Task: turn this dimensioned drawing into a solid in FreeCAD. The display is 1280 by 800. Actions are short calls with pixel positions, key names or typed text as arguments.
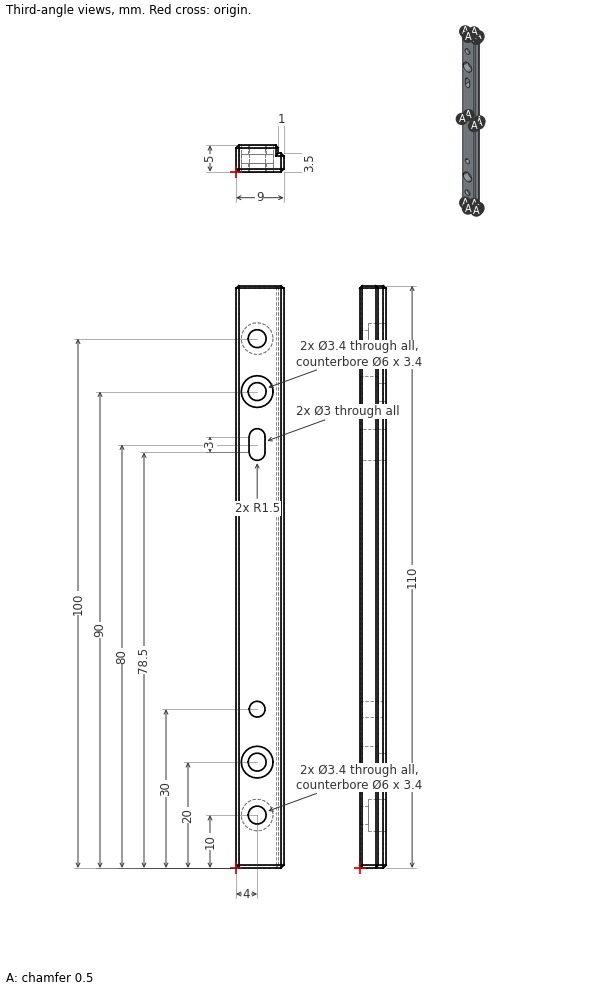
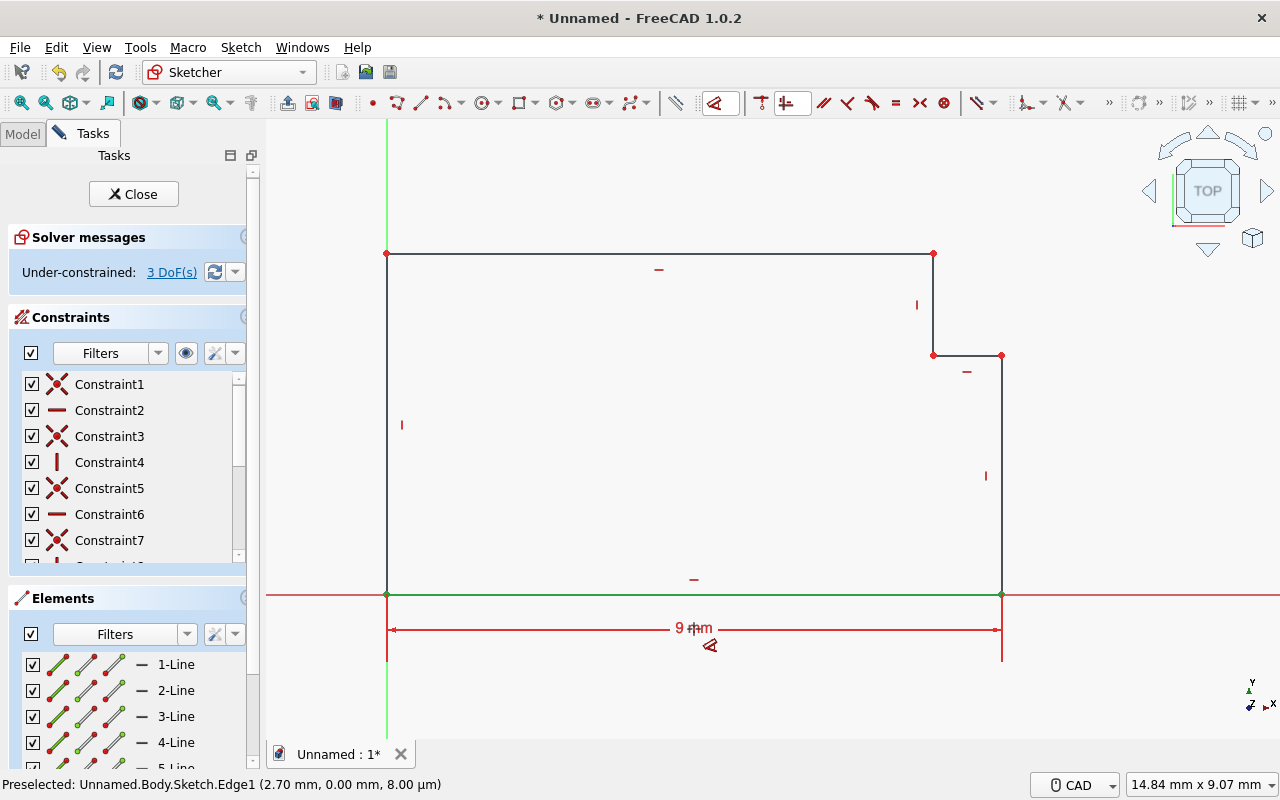
click(981, 356)
click(967, 322)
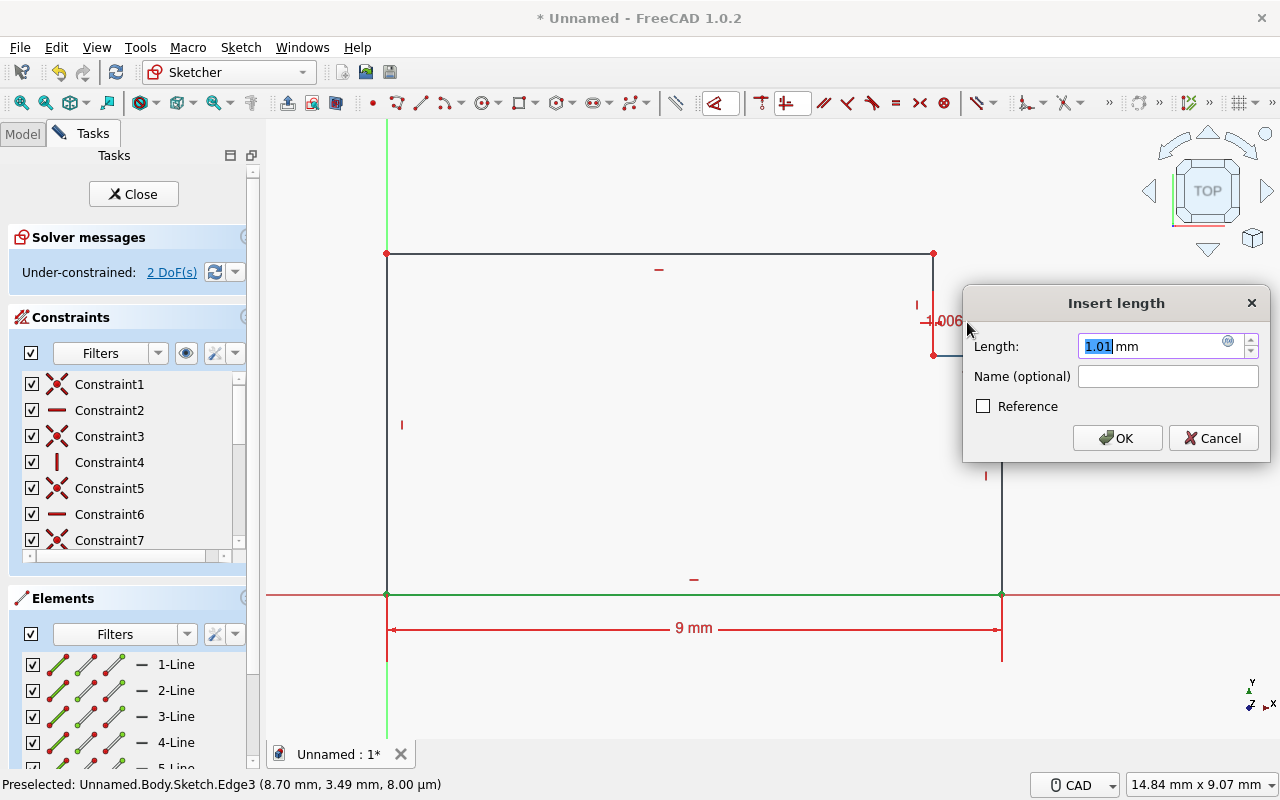
text(1)
key(Return)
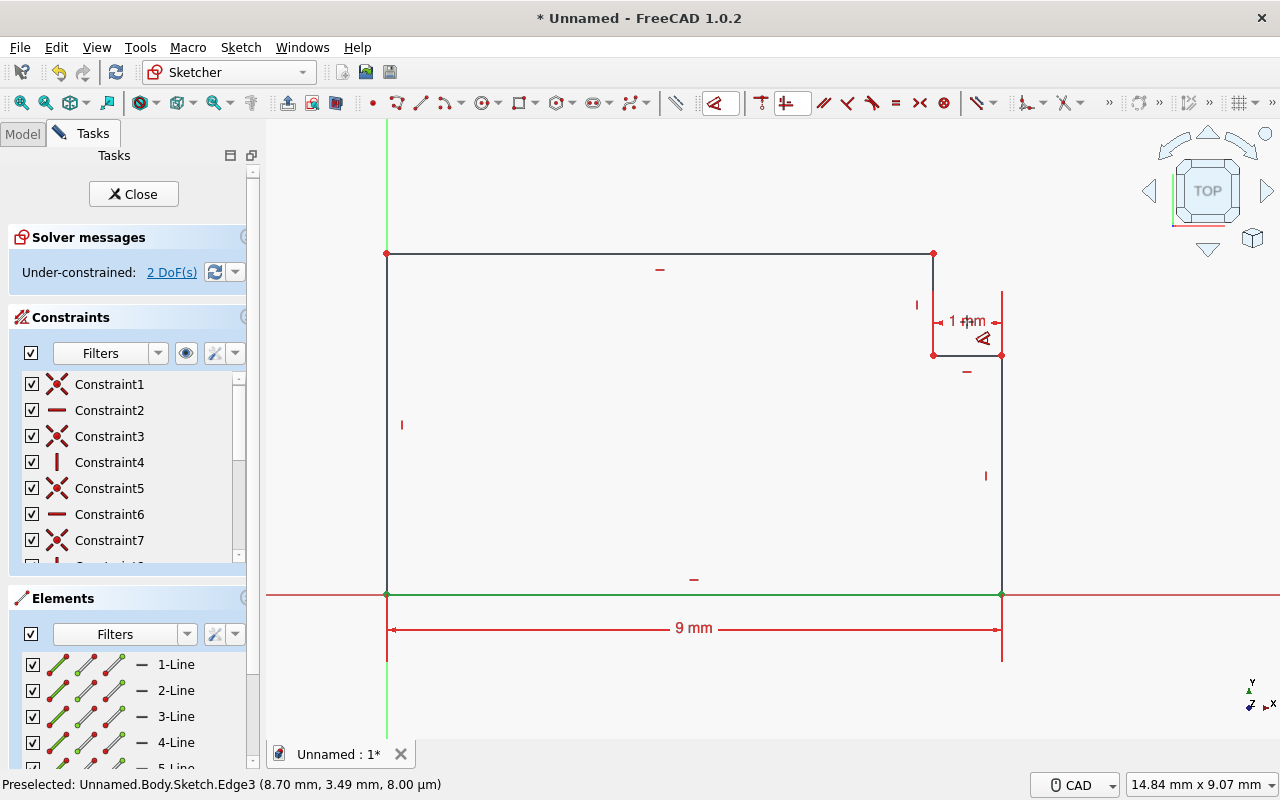
click(387, 356)
click(353, 424)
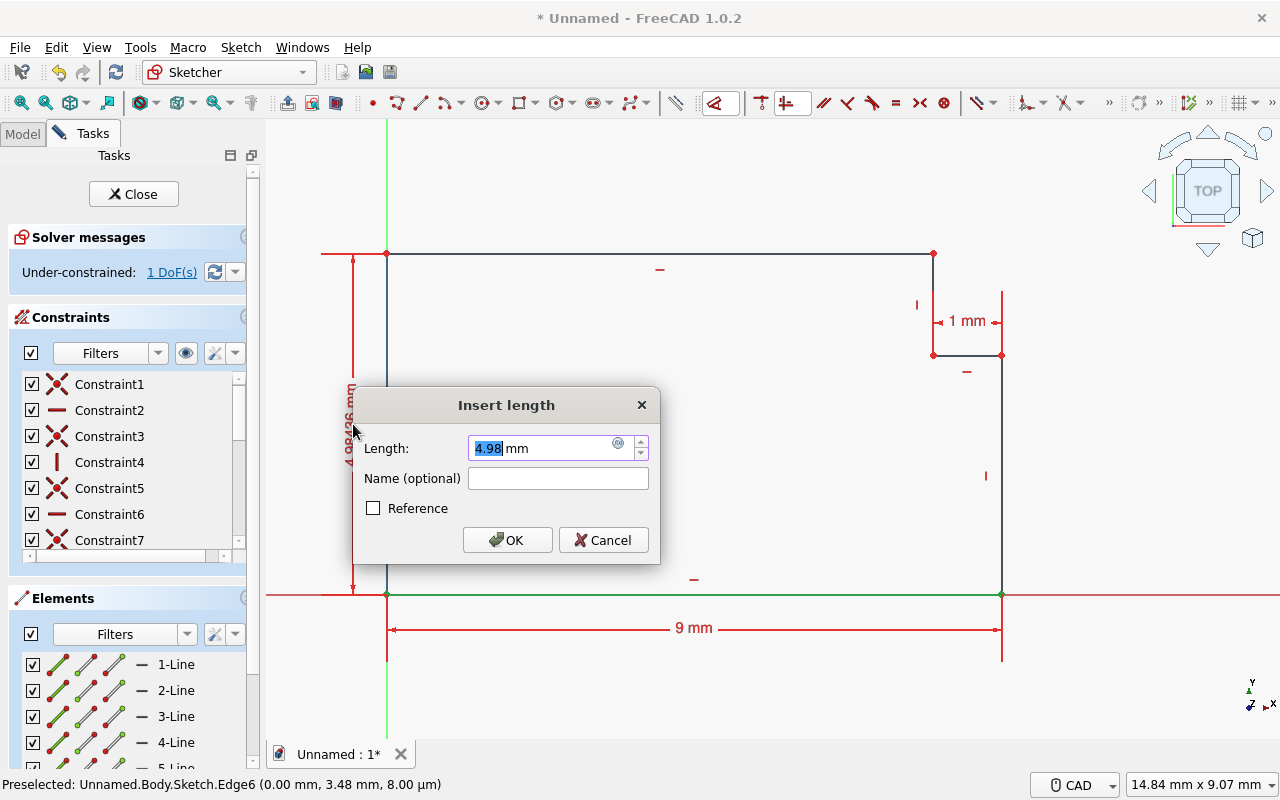
text(5)
key(Return)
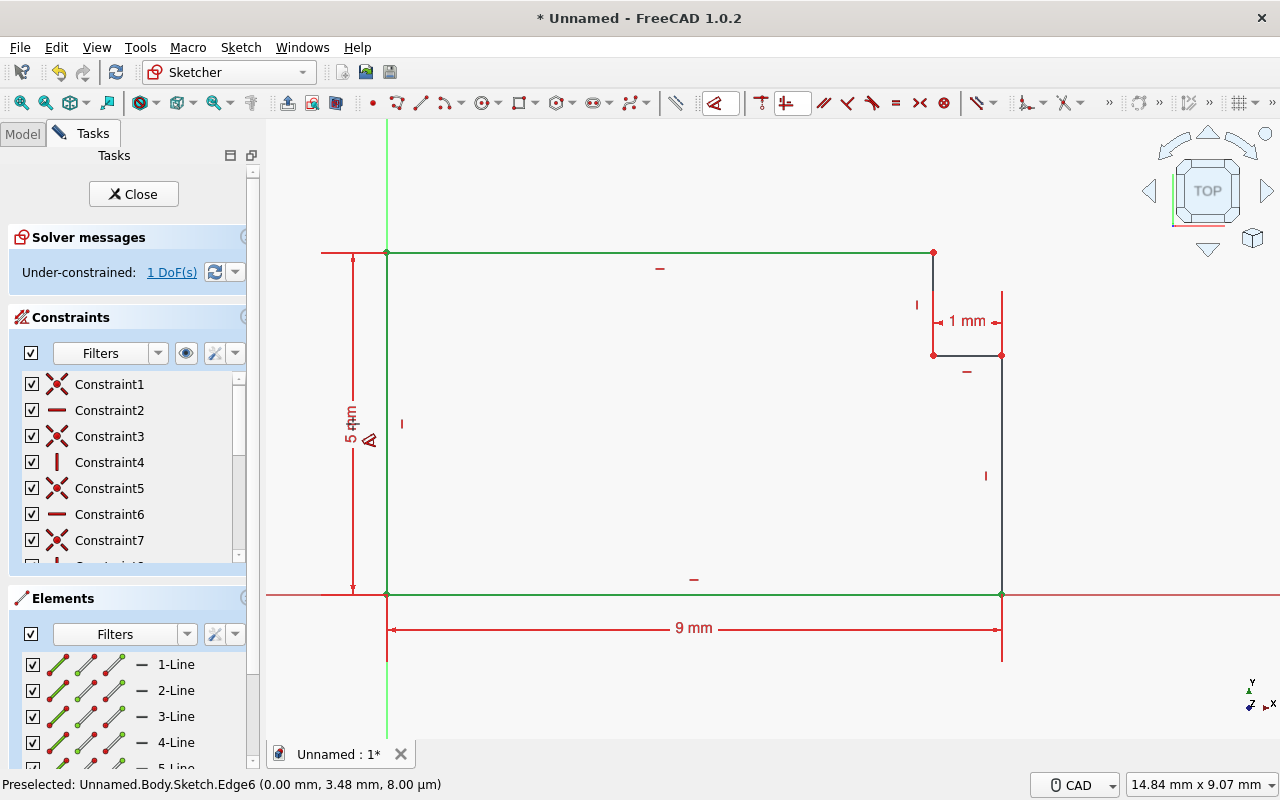
click(1002, 523)
click(1036, 475)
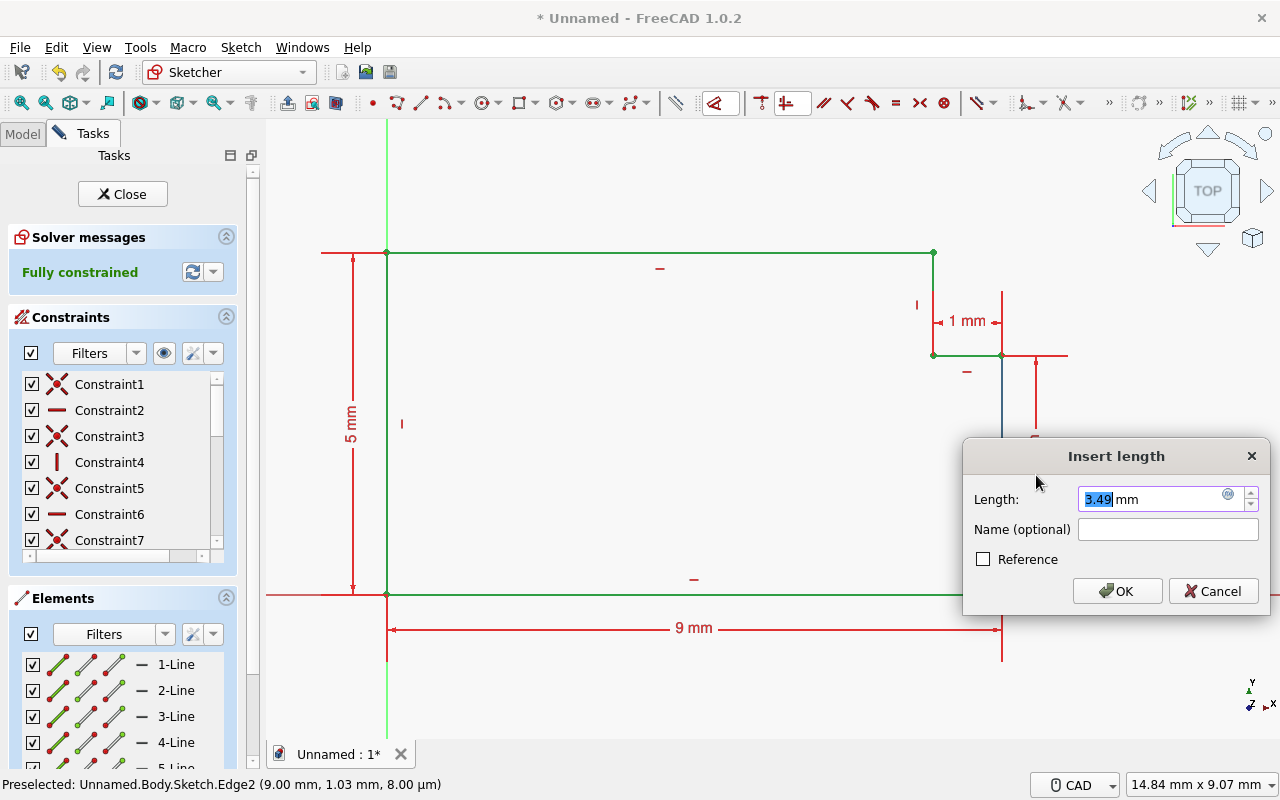
text(3.5)
key(Return)
key(Escape)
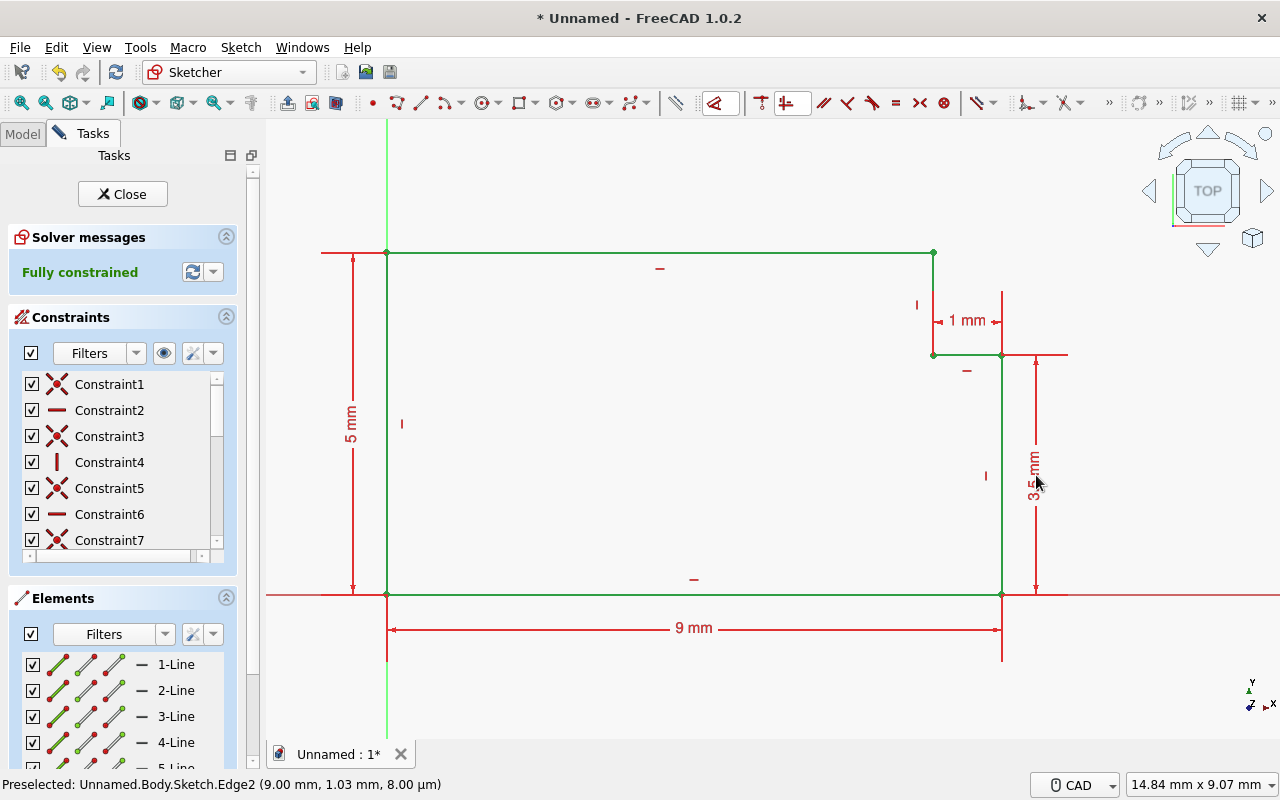
click(123, 194)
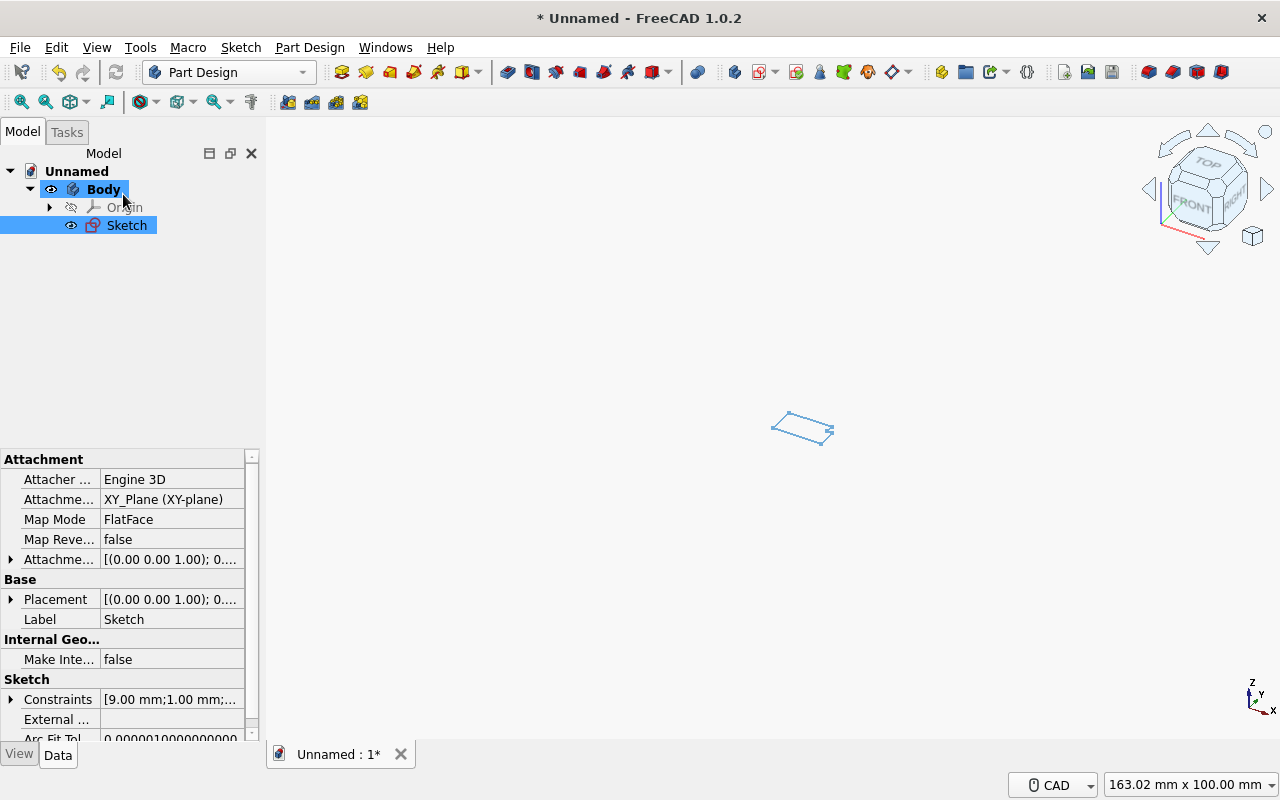
click(342, 72)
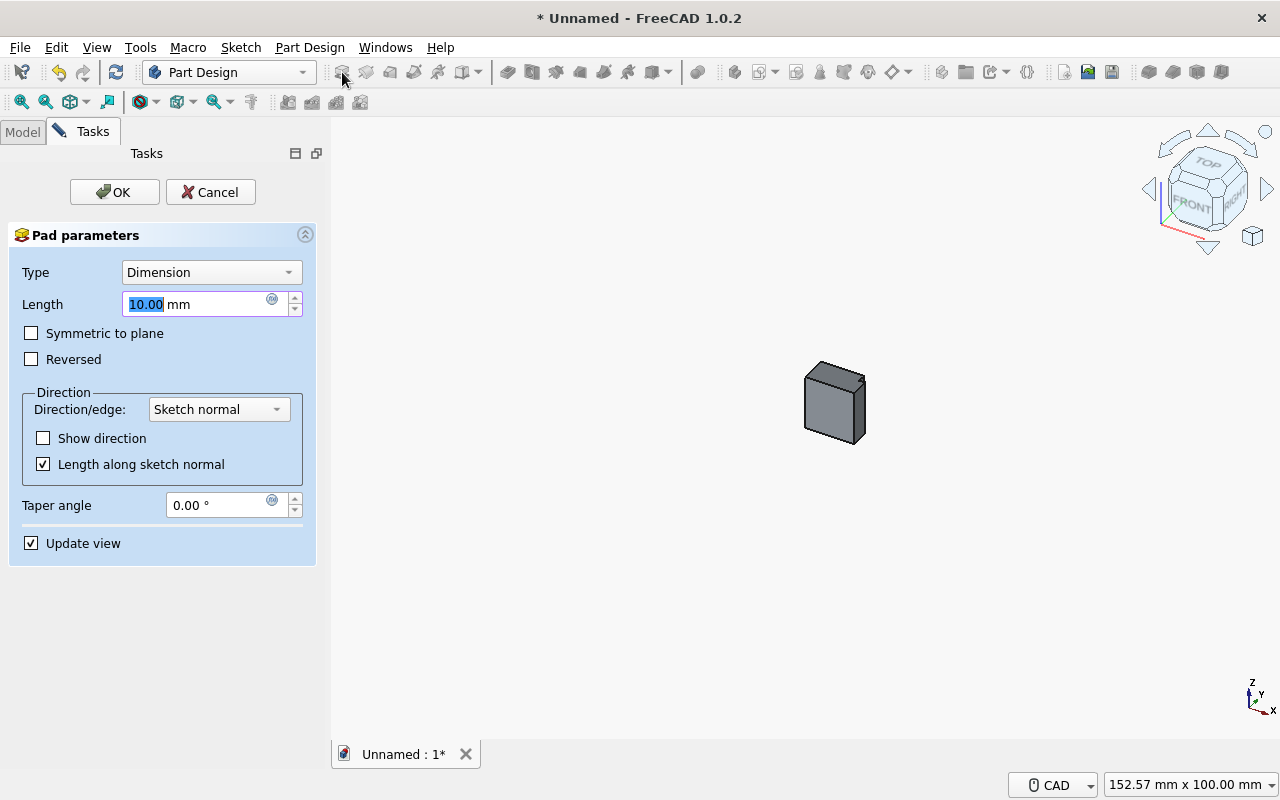
text(110)
key(Tab)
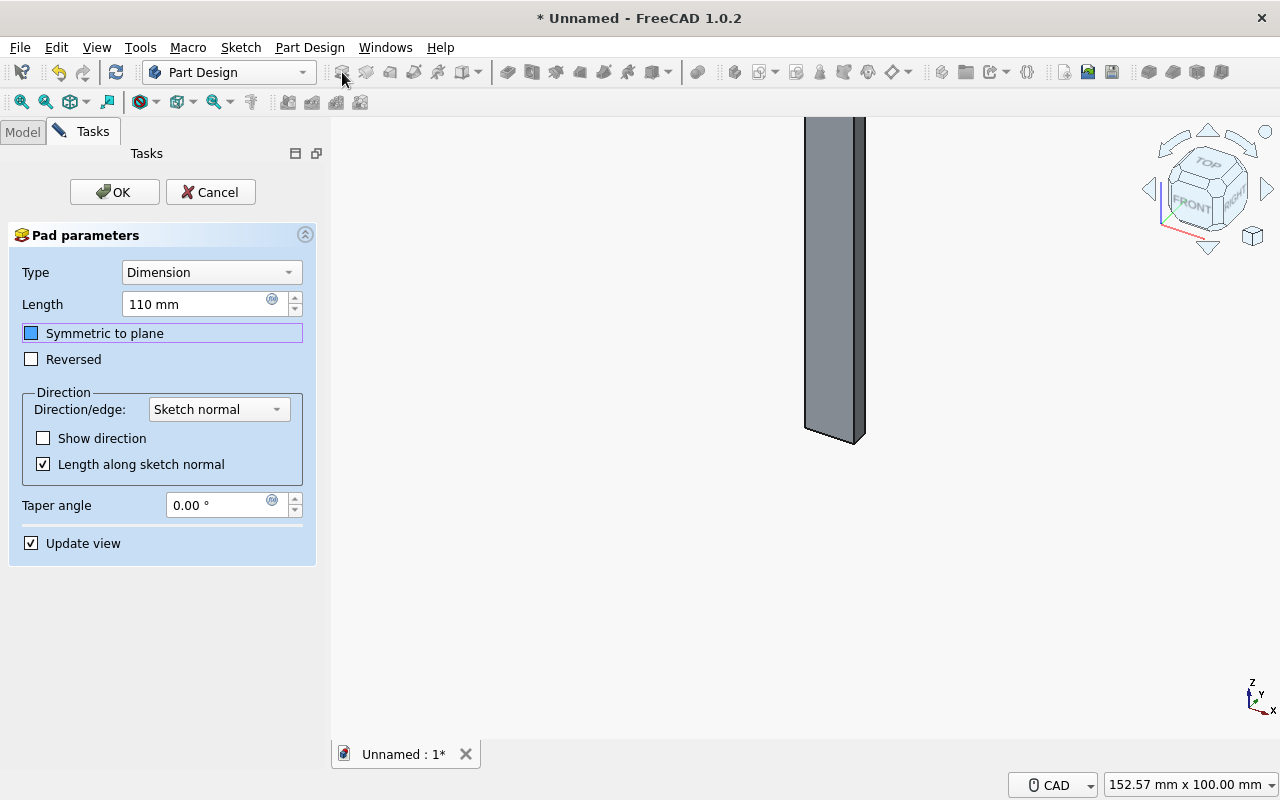
click(115, 192)